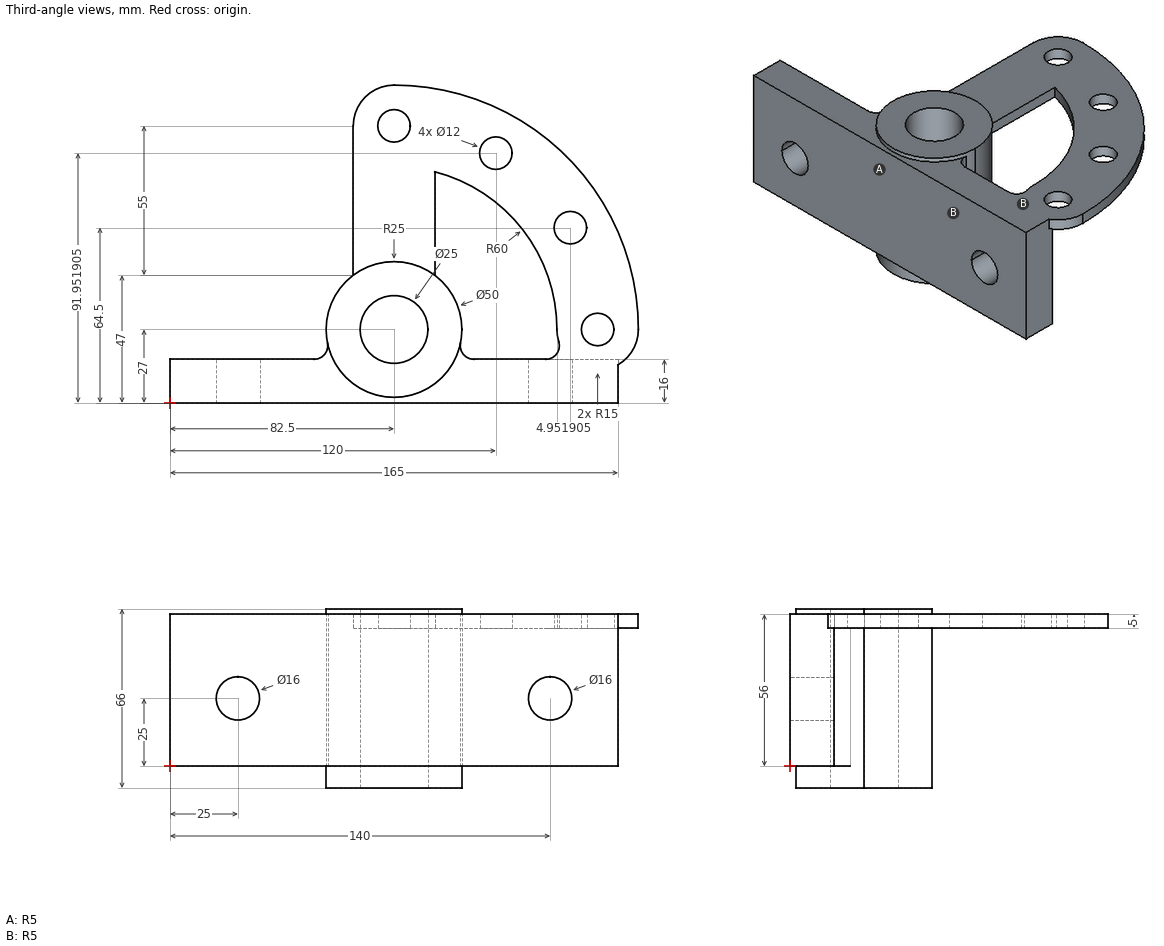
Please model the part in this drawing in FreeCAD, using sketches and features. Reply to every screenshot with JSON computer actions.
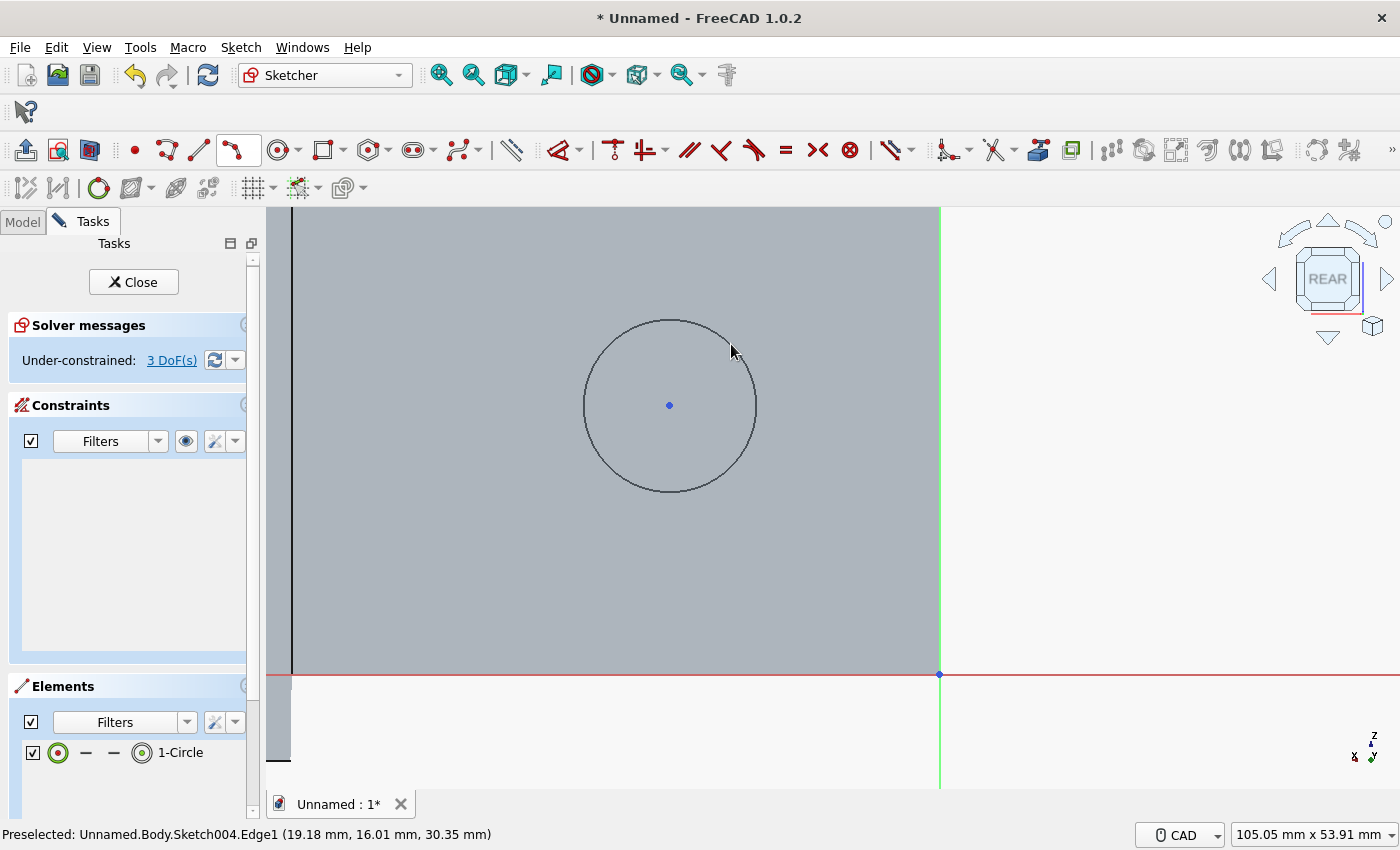
{"action": "left_click", "coordinate": [558, 150]}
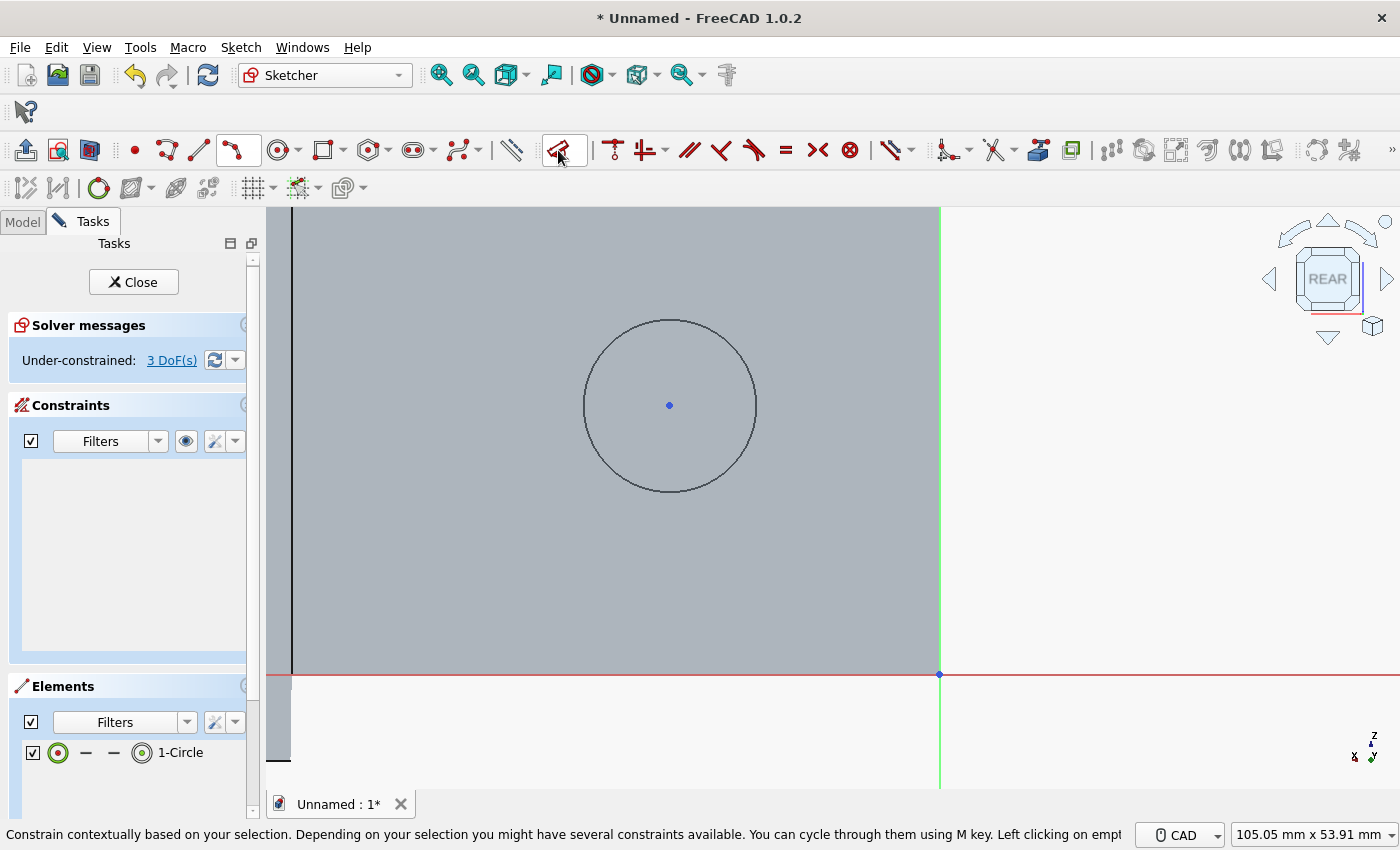
{"action": "left_click", "coordinate": [731, 345]}
{"action": "left_click", "coordinate": [754, 322]}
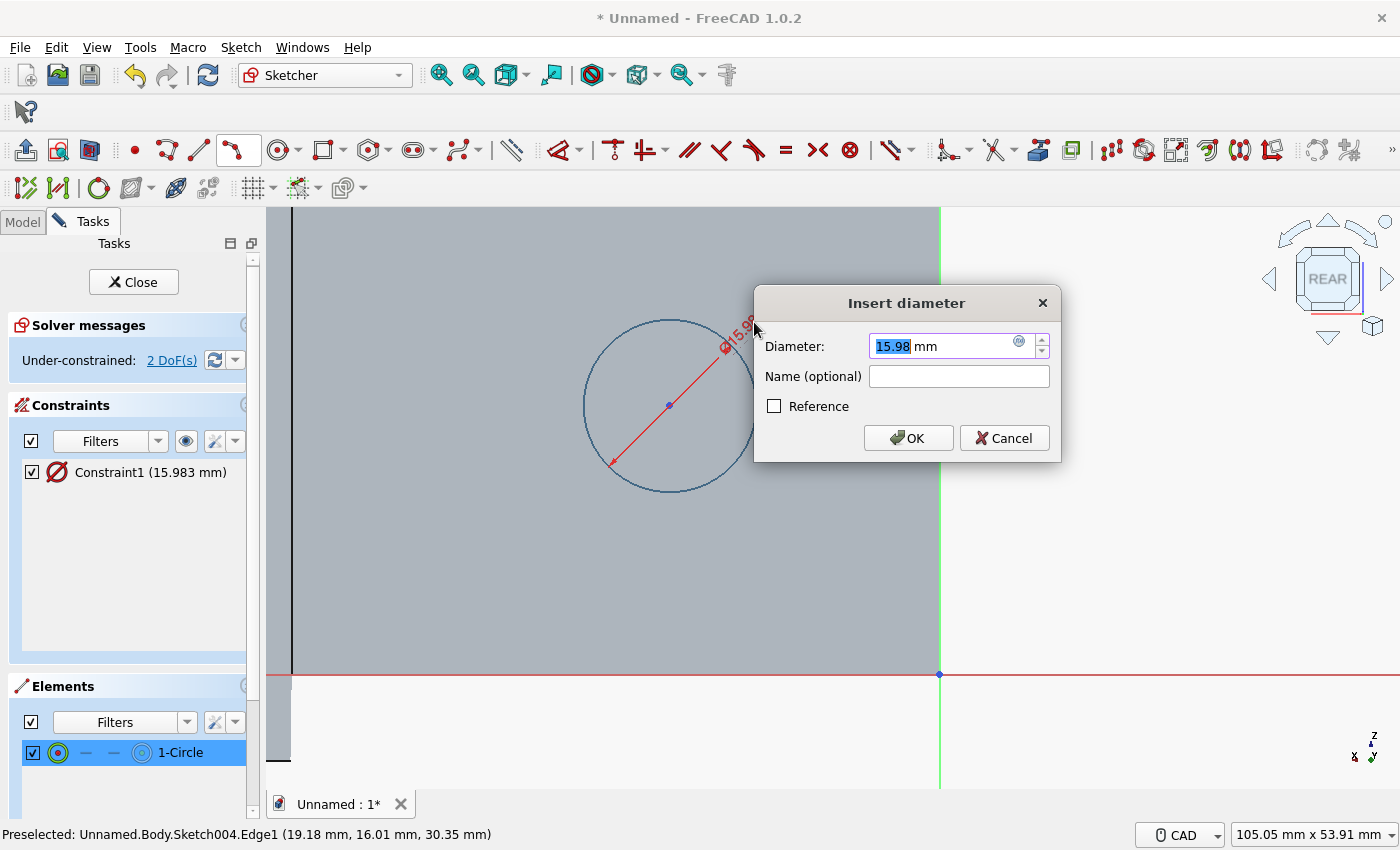
{"action": "type", "text": "16"}
{"action": "key", "text": "Return"}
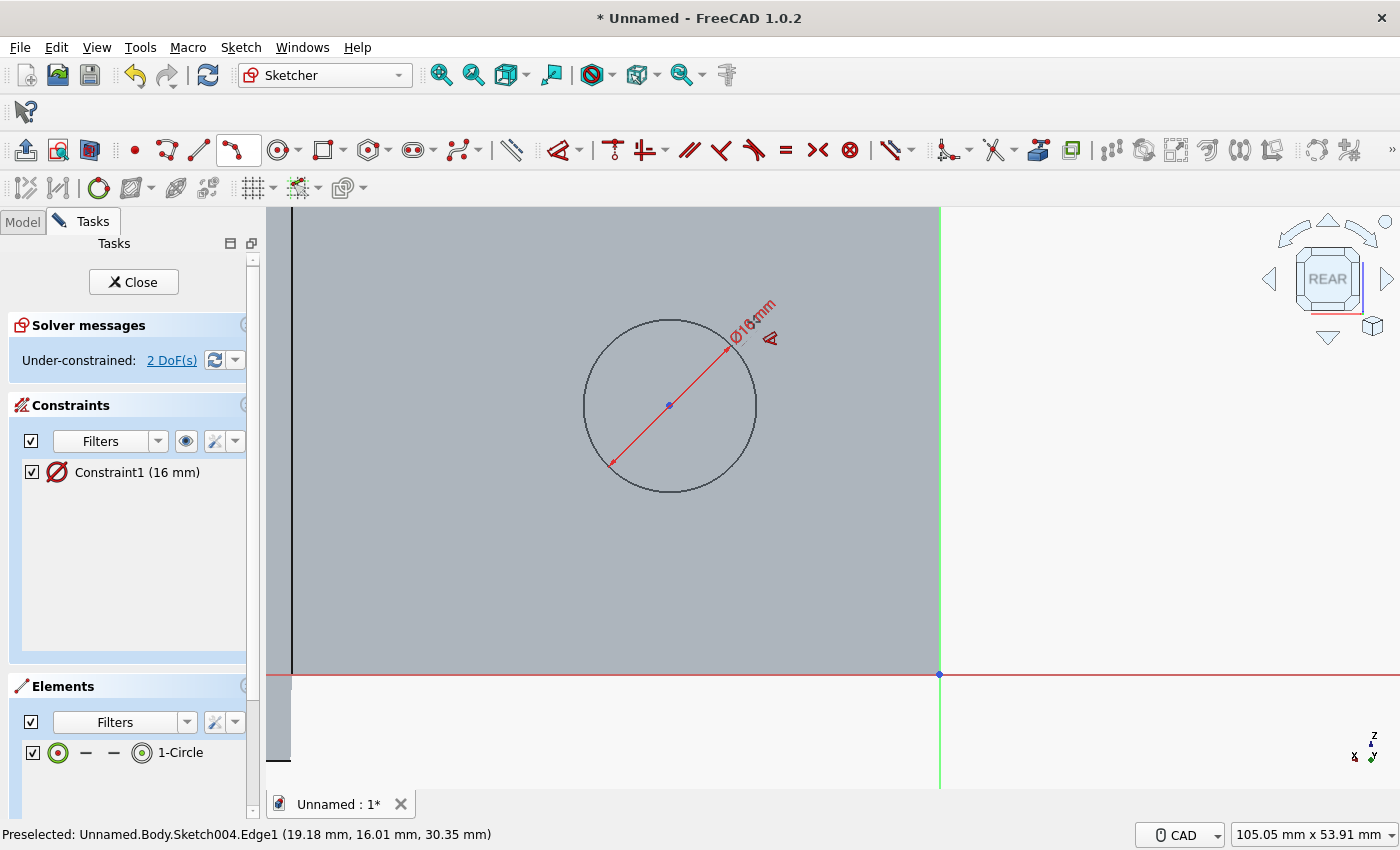
{"action": "left_click", "coordinate": [670, 406]}
{"action": "left_click", "coordinate": [805, 709]}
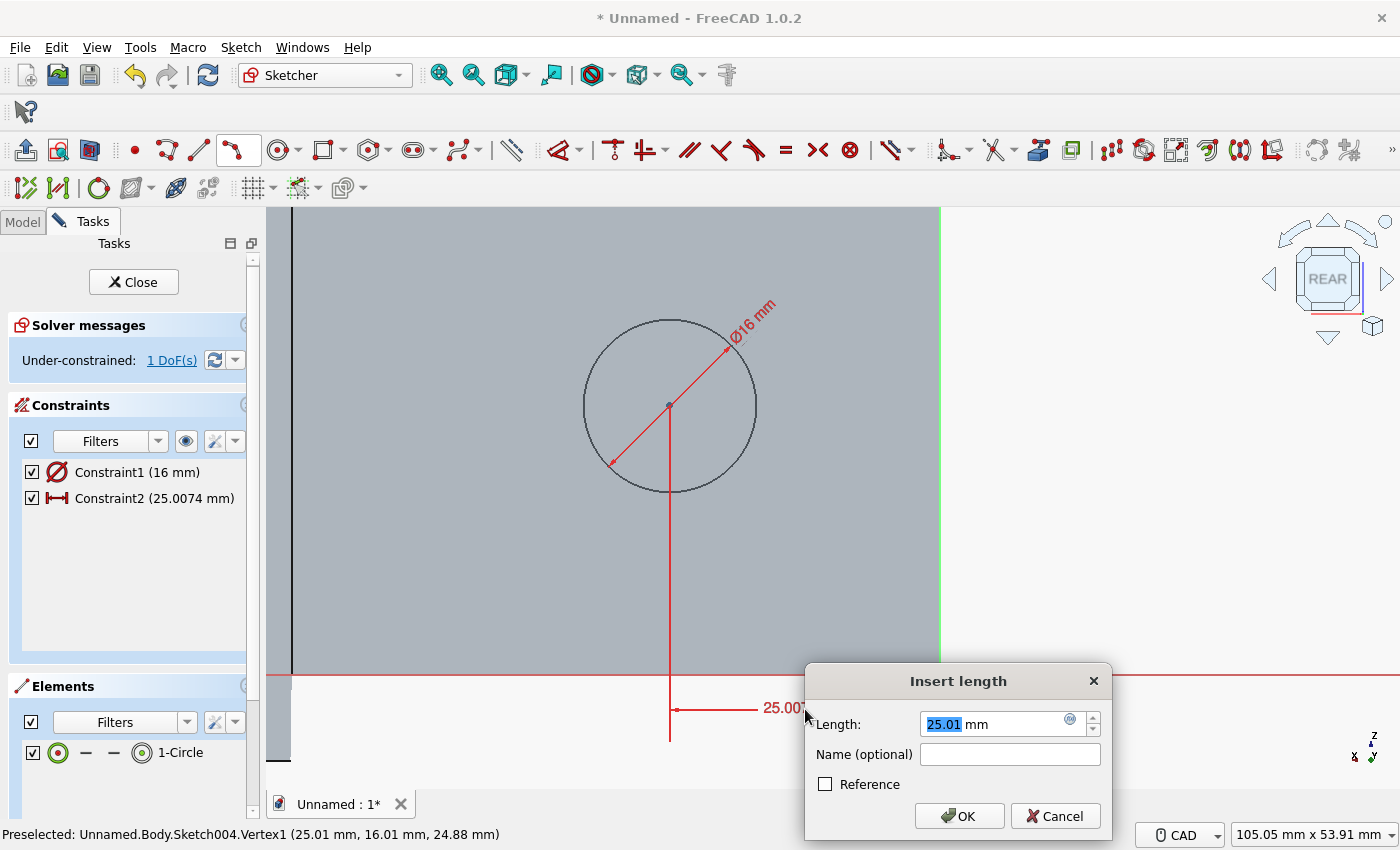
{"action": "type", "text": "25"}
{"action": "key", "text": "Return"}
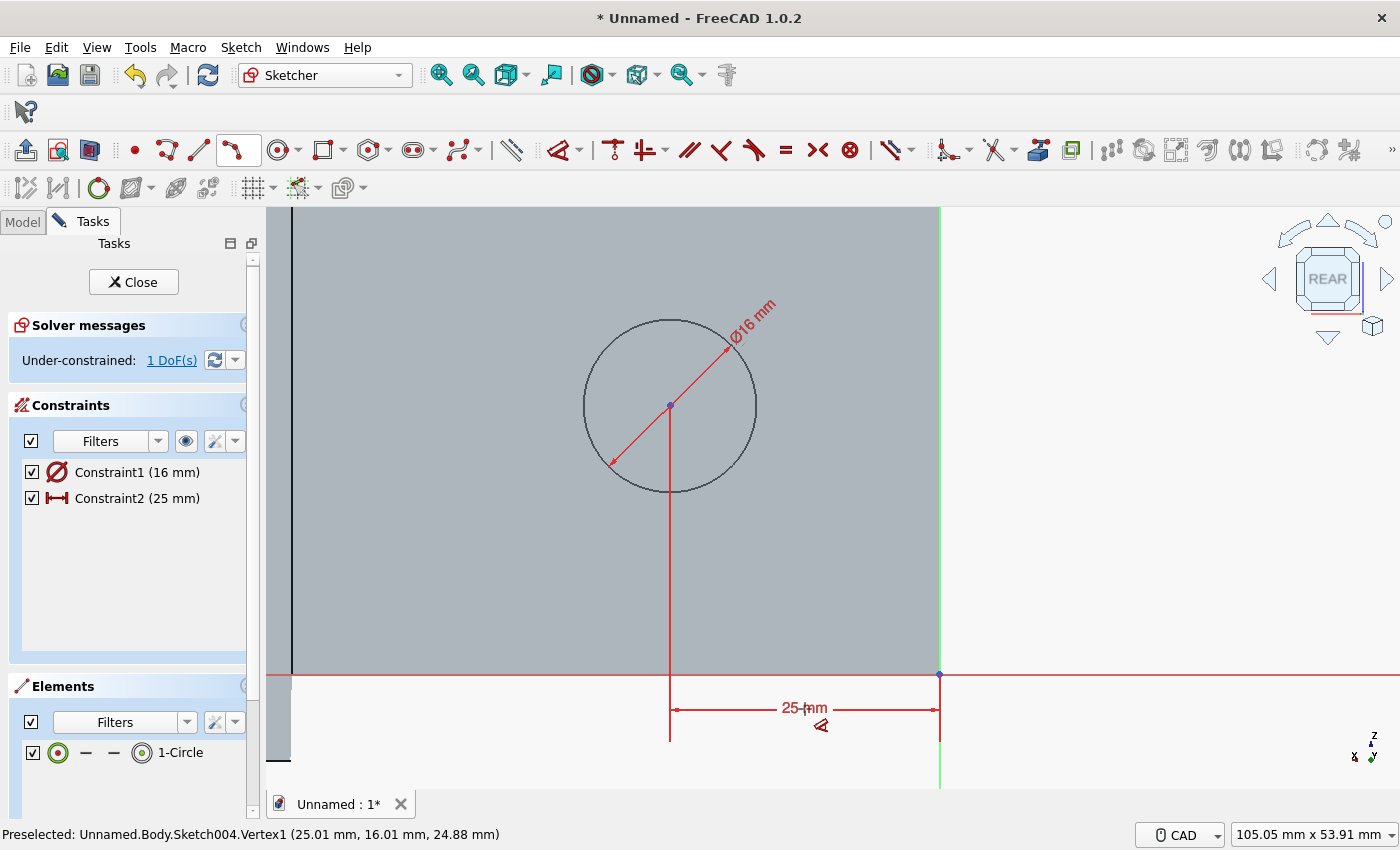
{"action": "left_click", "coordinate": [670, 406]}
{"action": "left_click", "coordinate": [974, 540]}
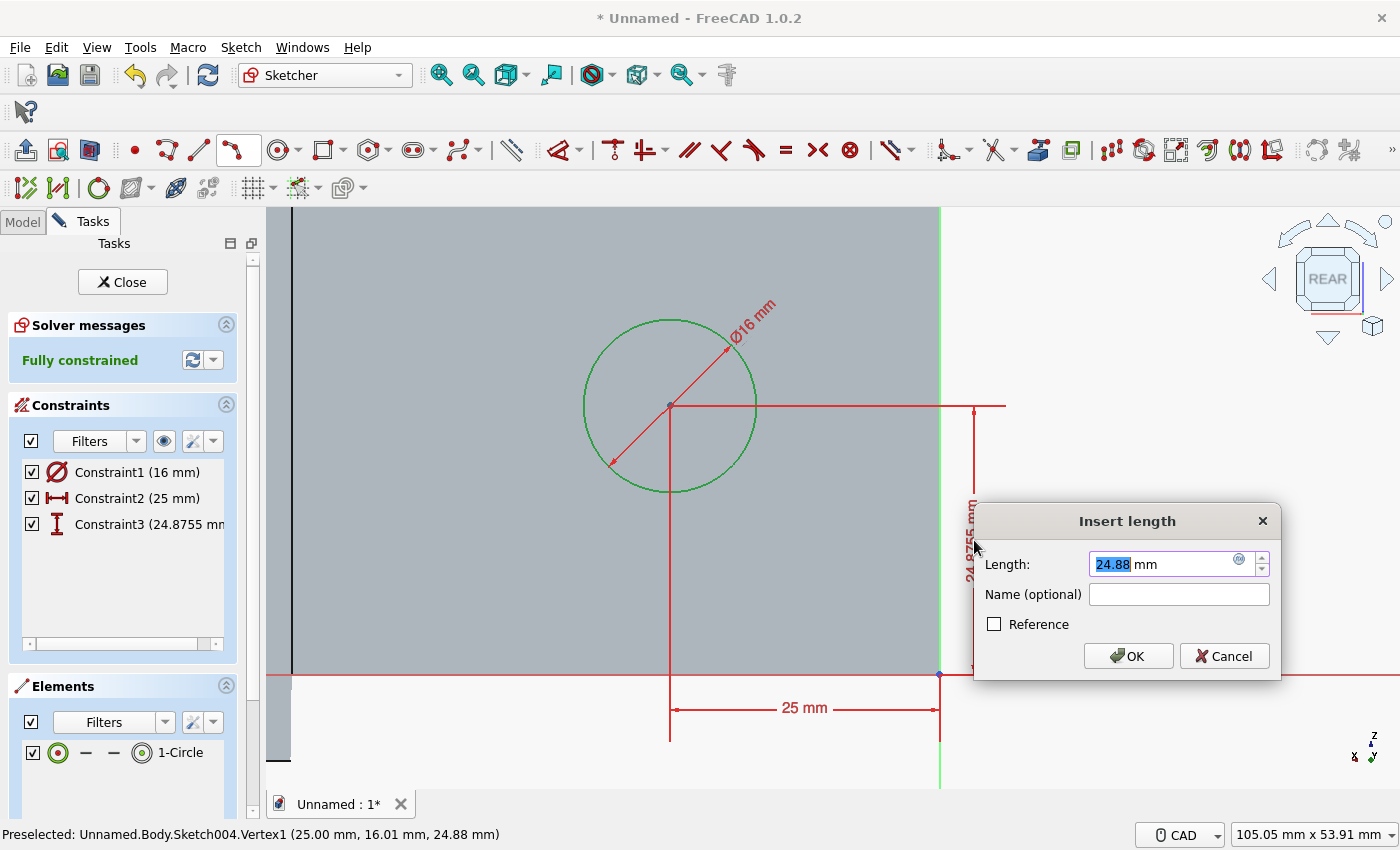
{"action": "type", "text": "25"}
{"action": "key", "text": "Return"}
{"action": "key", "text": "Escape"}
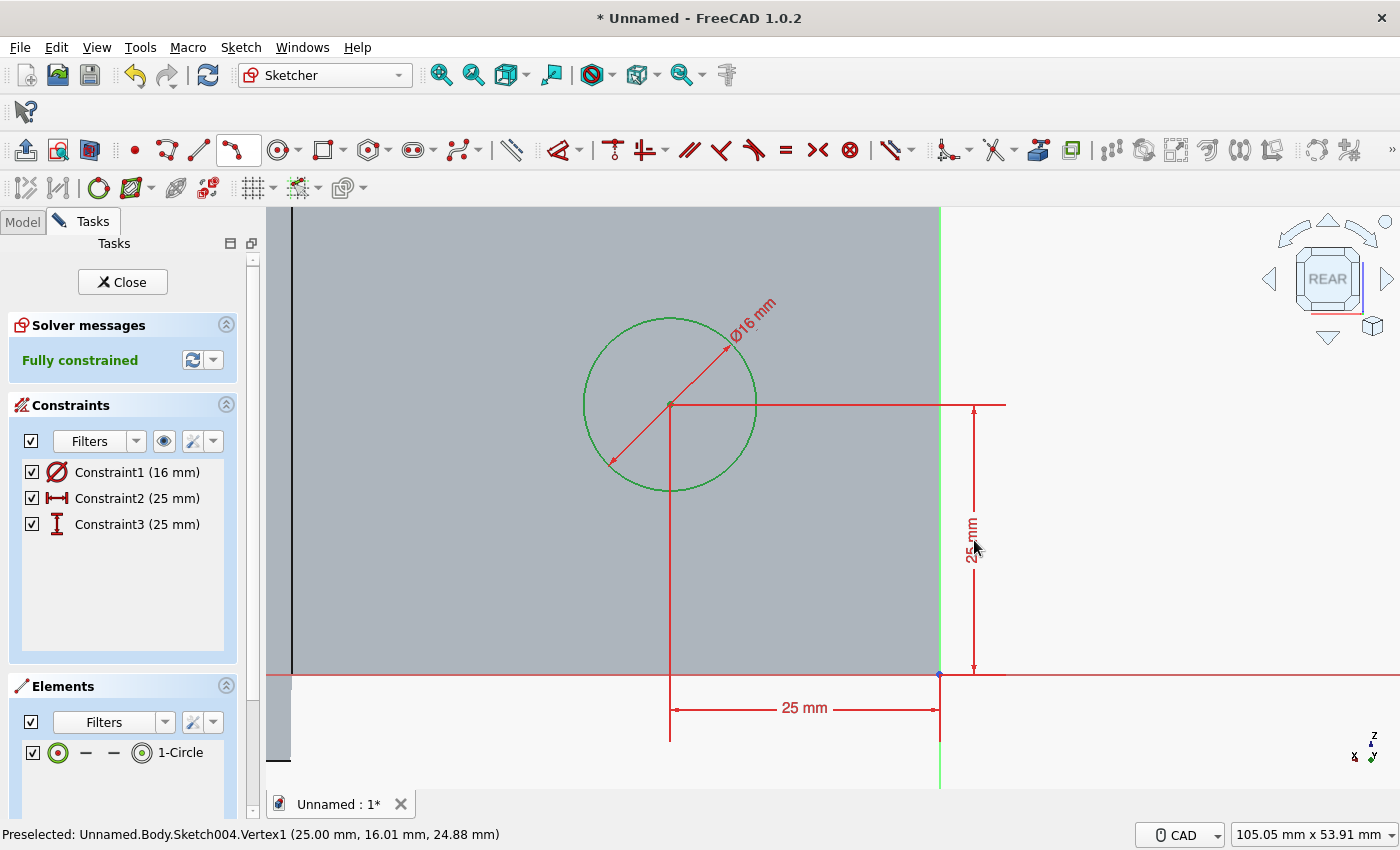
{"action": "left_click", "coordinate": [123, 282]}